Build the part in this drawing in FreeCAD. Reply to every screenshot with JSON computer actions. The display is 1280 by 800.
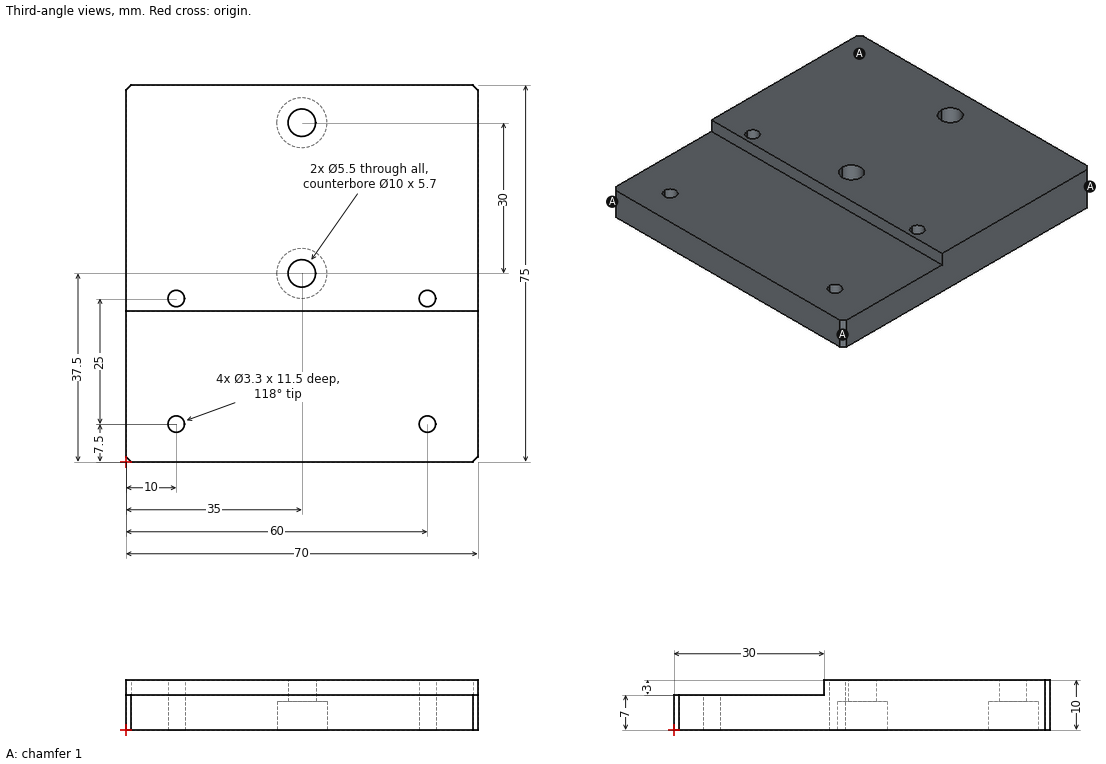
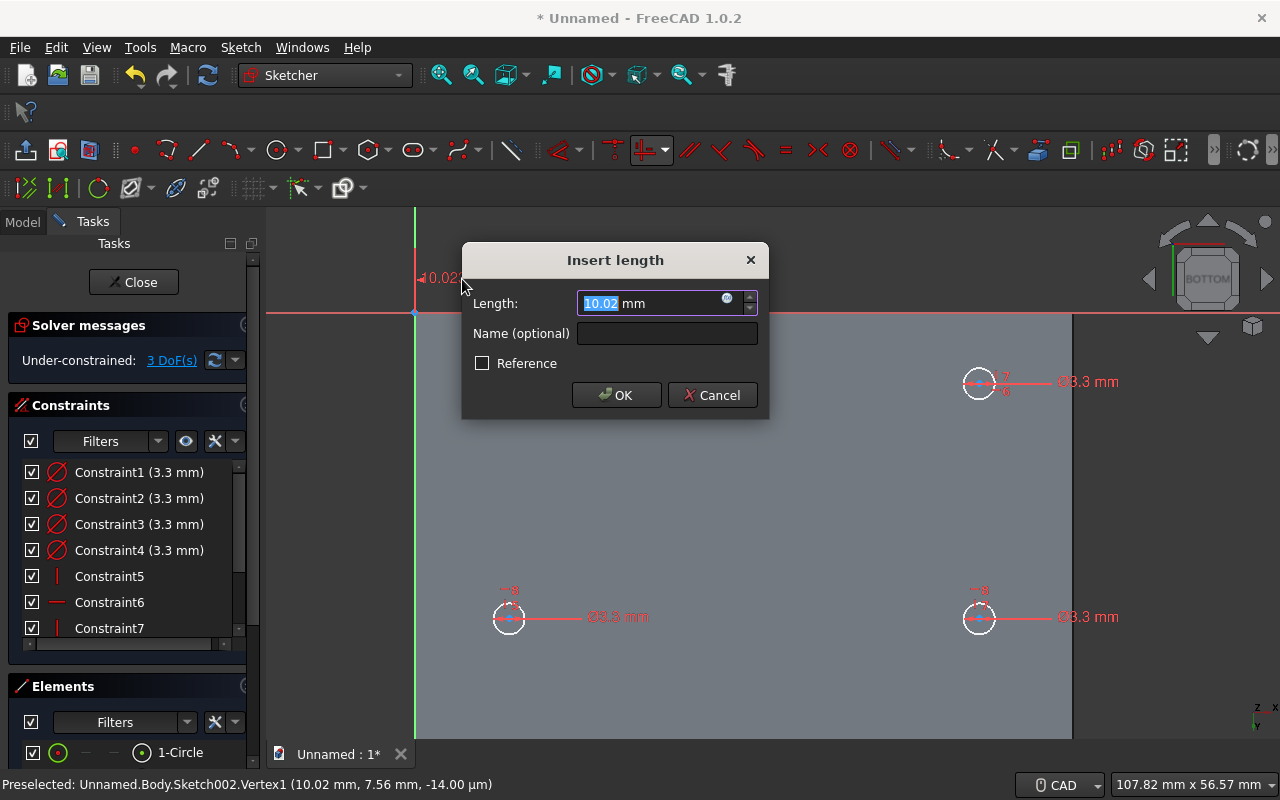
{"action": "type", "text": "10"}
{"action": "key", "text": "Return"}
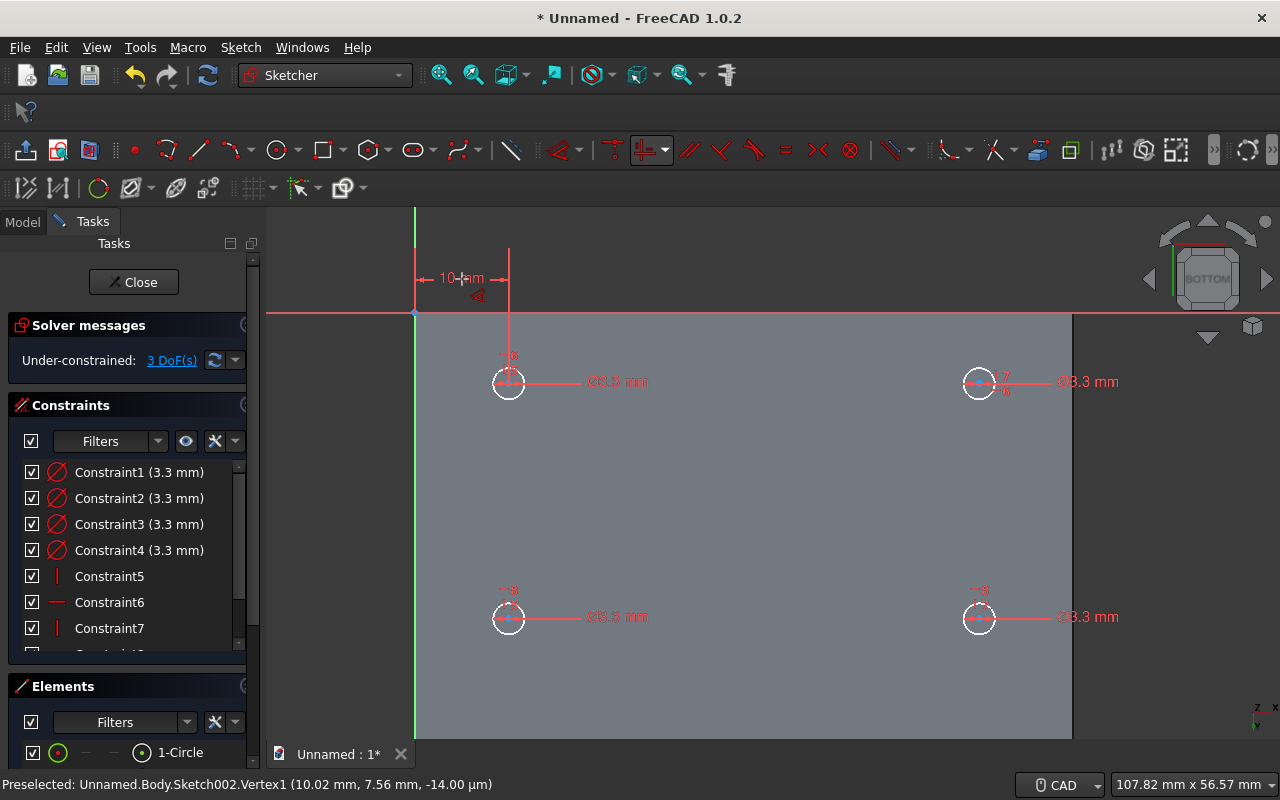
{"action": "left_click", "coordinate": [979, 384]}
{"action": "left_click", "coordinate": [697, 279]}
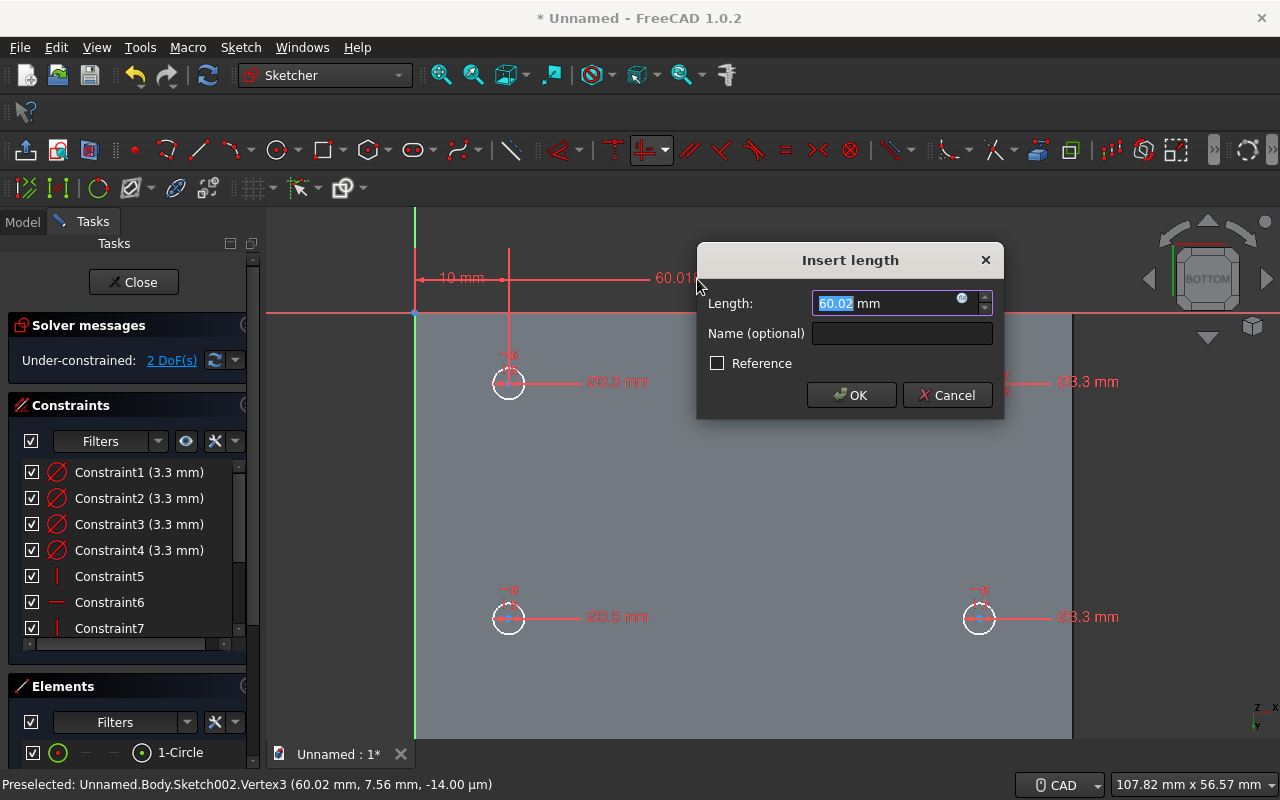
{"action": "type", "text": "60"}
{"action": "key", "text": "Return"}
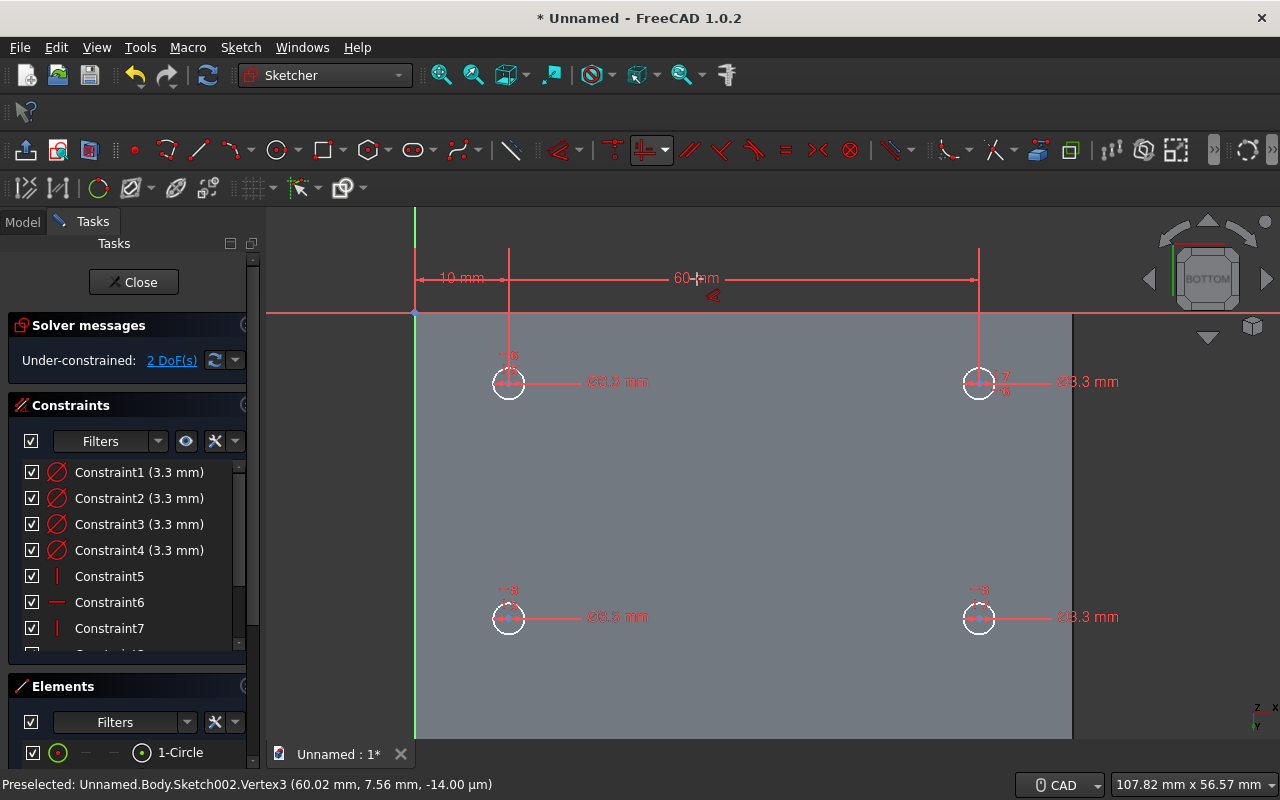
{"action": "left_click", "coordinate": [509, 384]}
{"action": "left_click", "coordinate": [381, 348]}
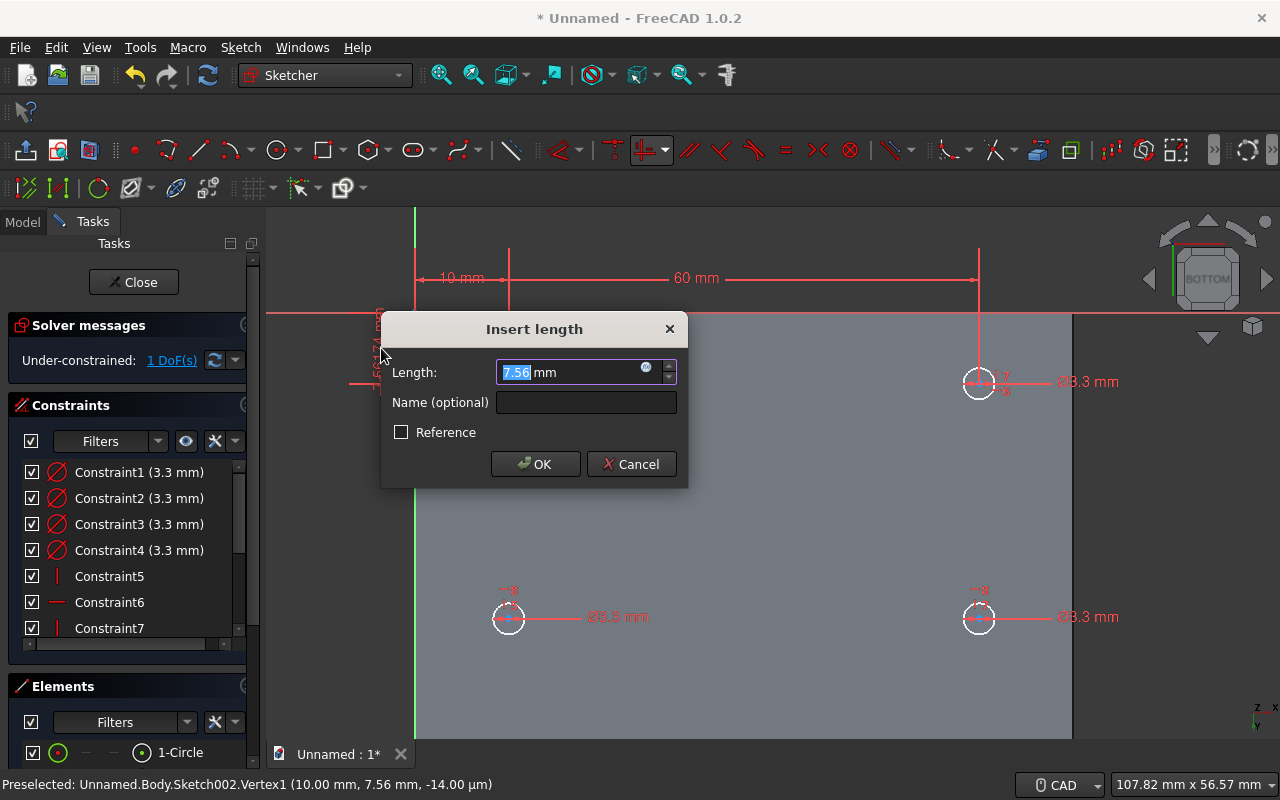
{"action": "type", "text": "7.5"}
{"action": "key", "text": "Return"}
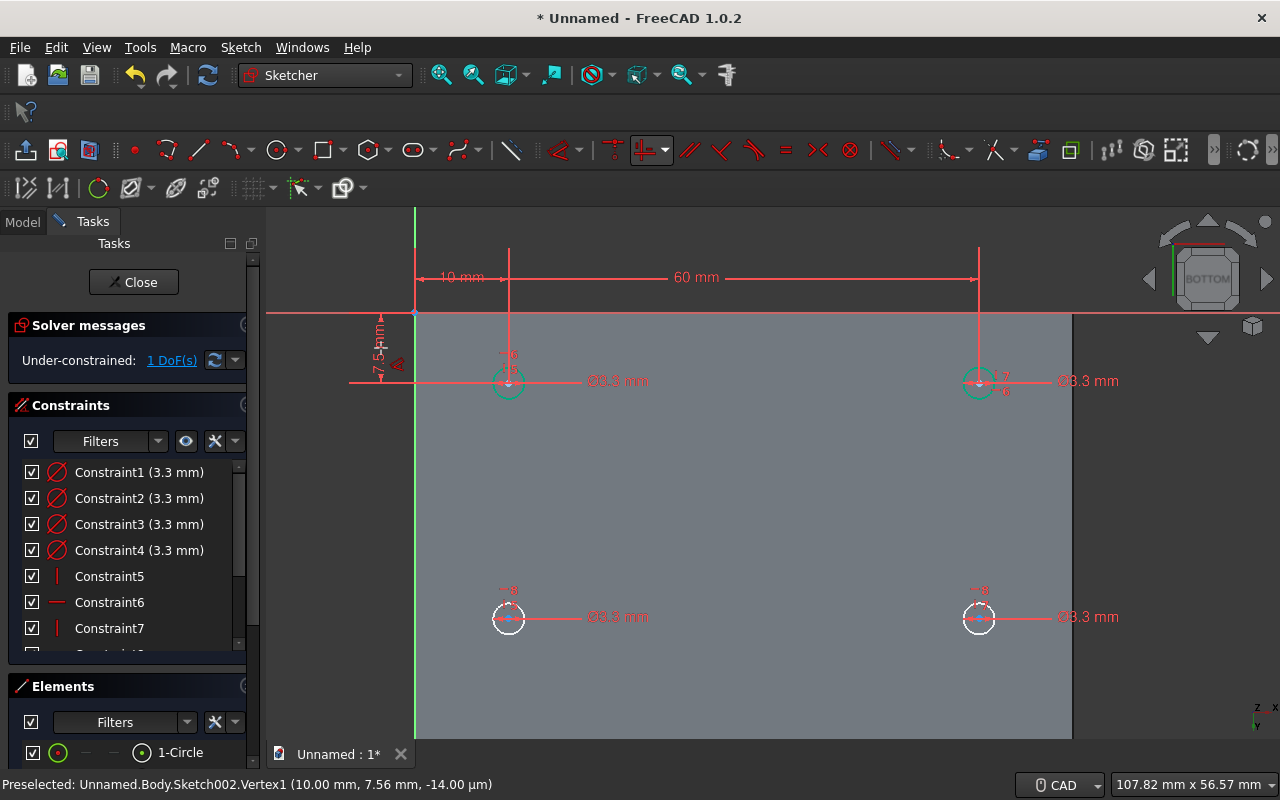
{"action": "left_click", "coordinate": [509, 383]}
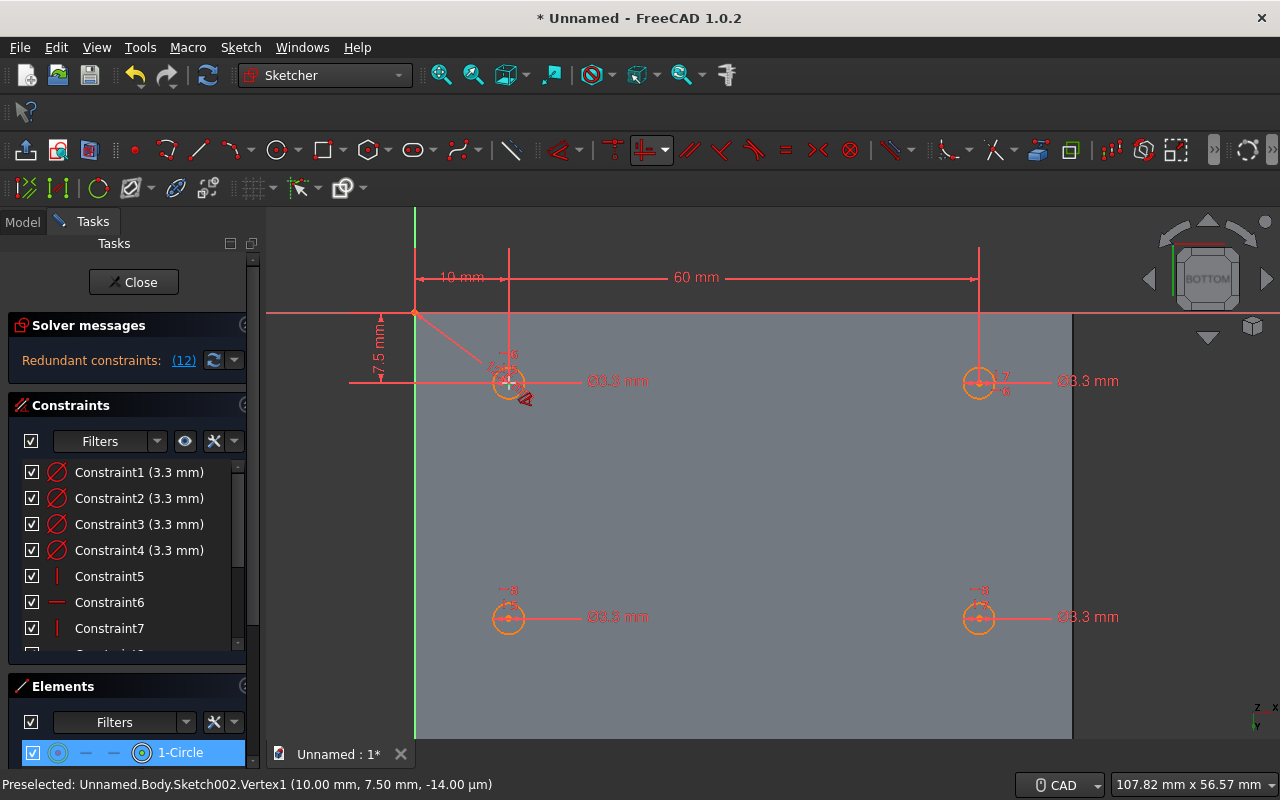
{"action": "left_click", "coordinate": [509, 619]}
{"action": "left_click", "coordinate": [475, 501]}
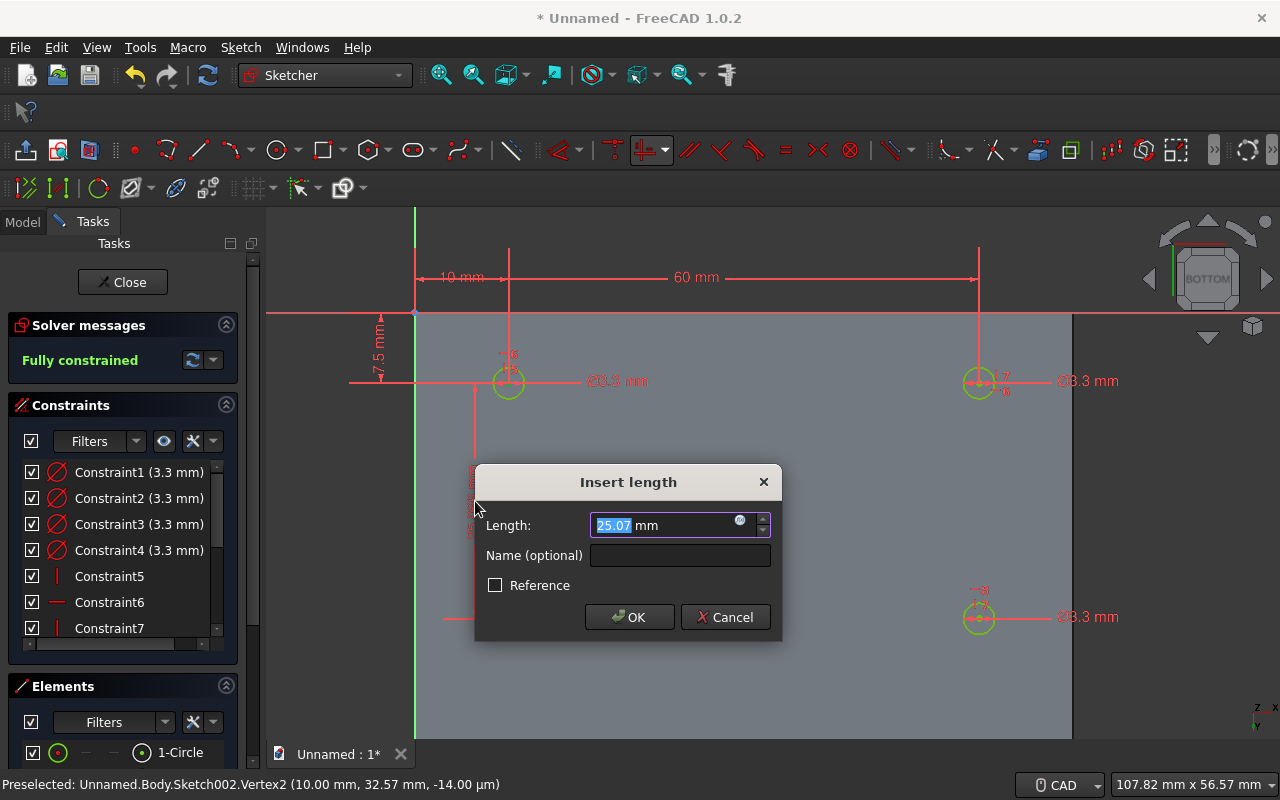
{"action": "type", "text": "25"}
{"action": "key", "text": "Return"}
{"action": "key", "text": "Escape"}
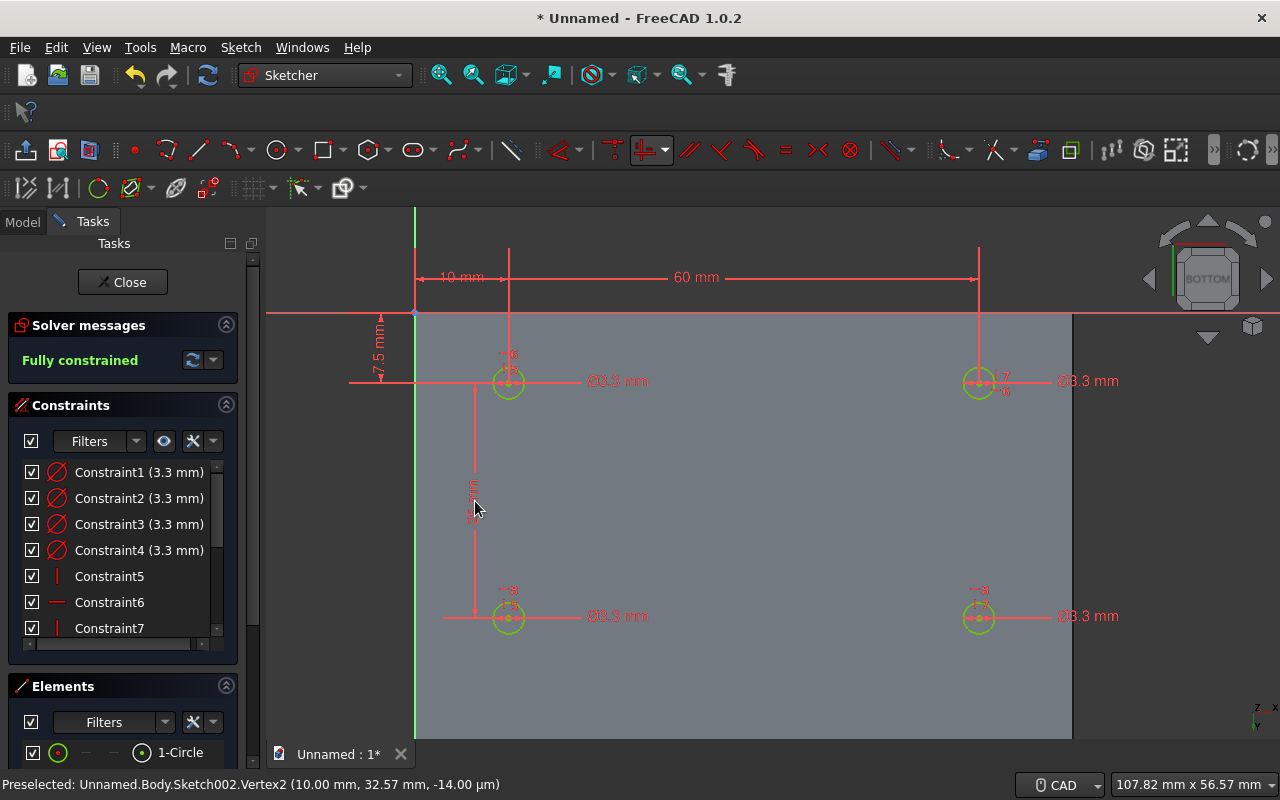
{"action": "left_click", "coordinate": [123, 282]}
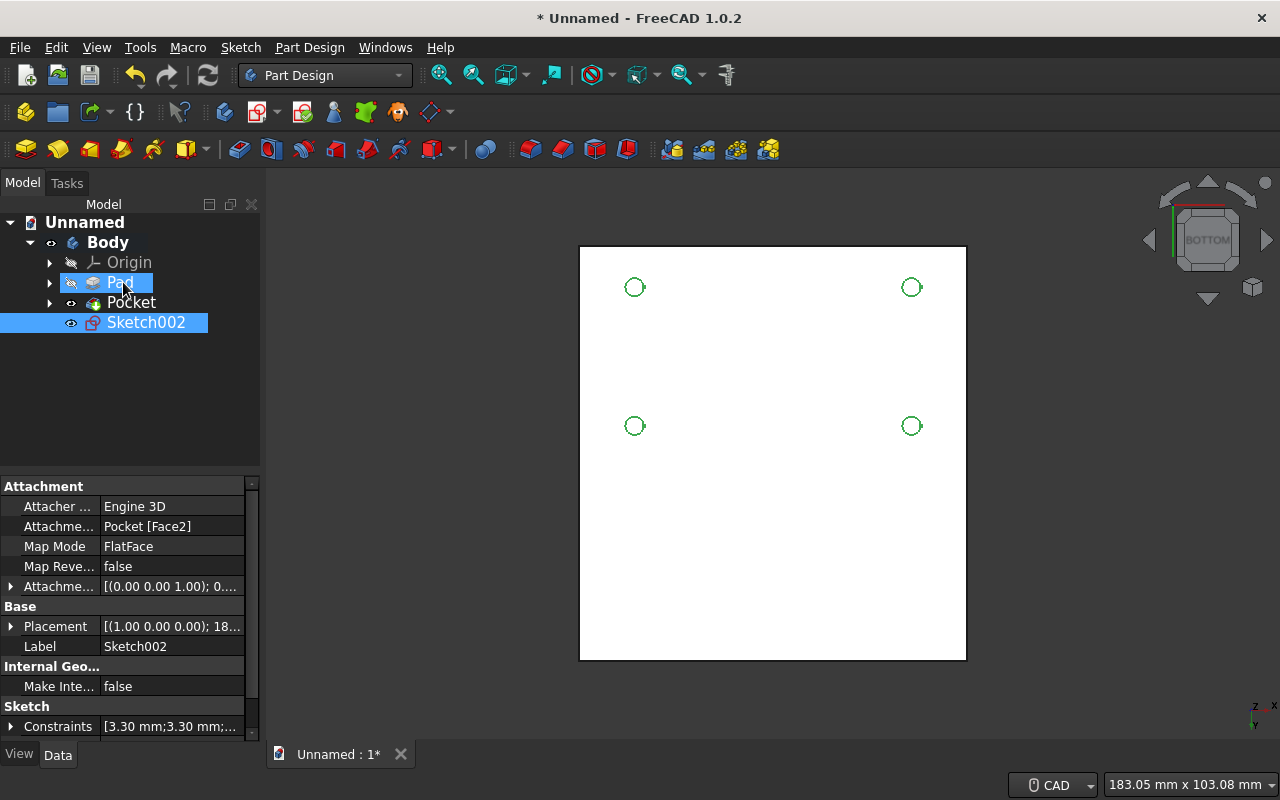
{"action": "left_click", "coordinate": [272, 150]}